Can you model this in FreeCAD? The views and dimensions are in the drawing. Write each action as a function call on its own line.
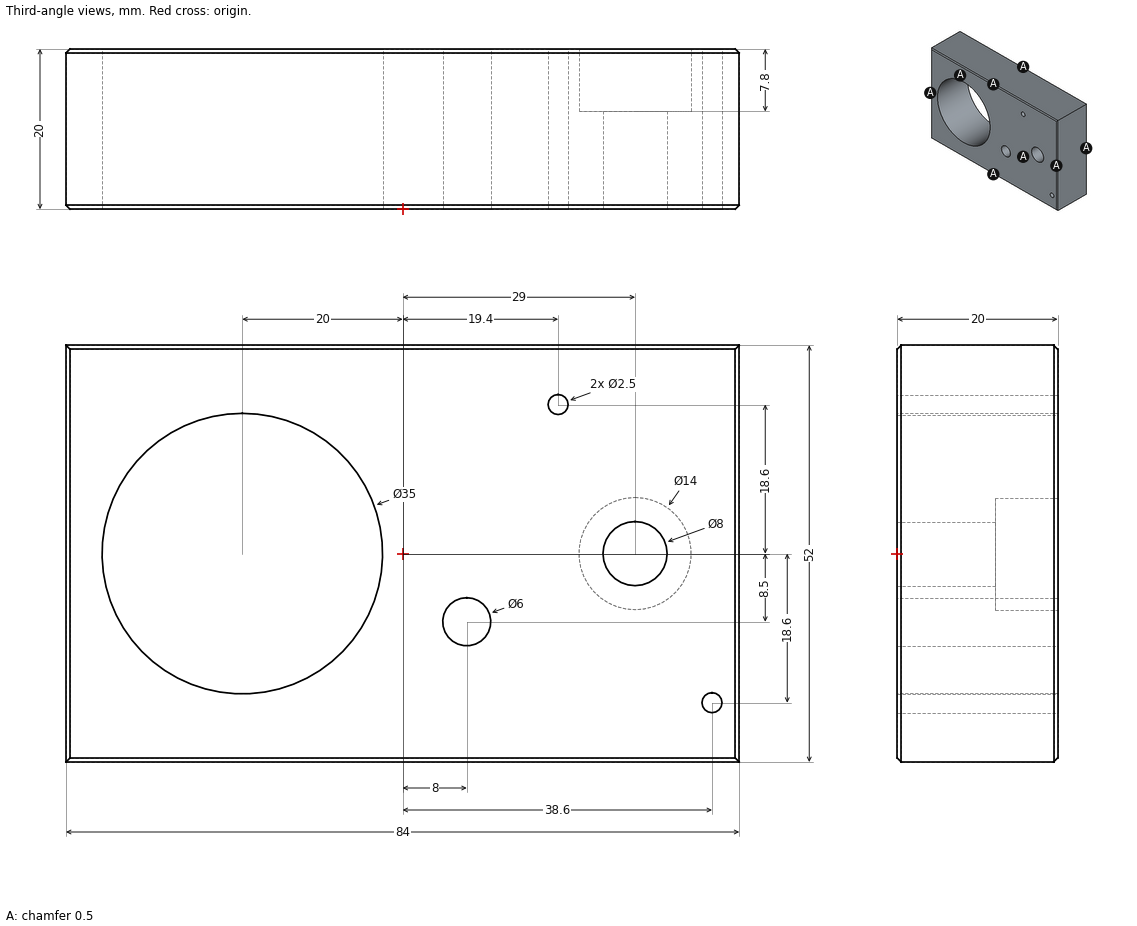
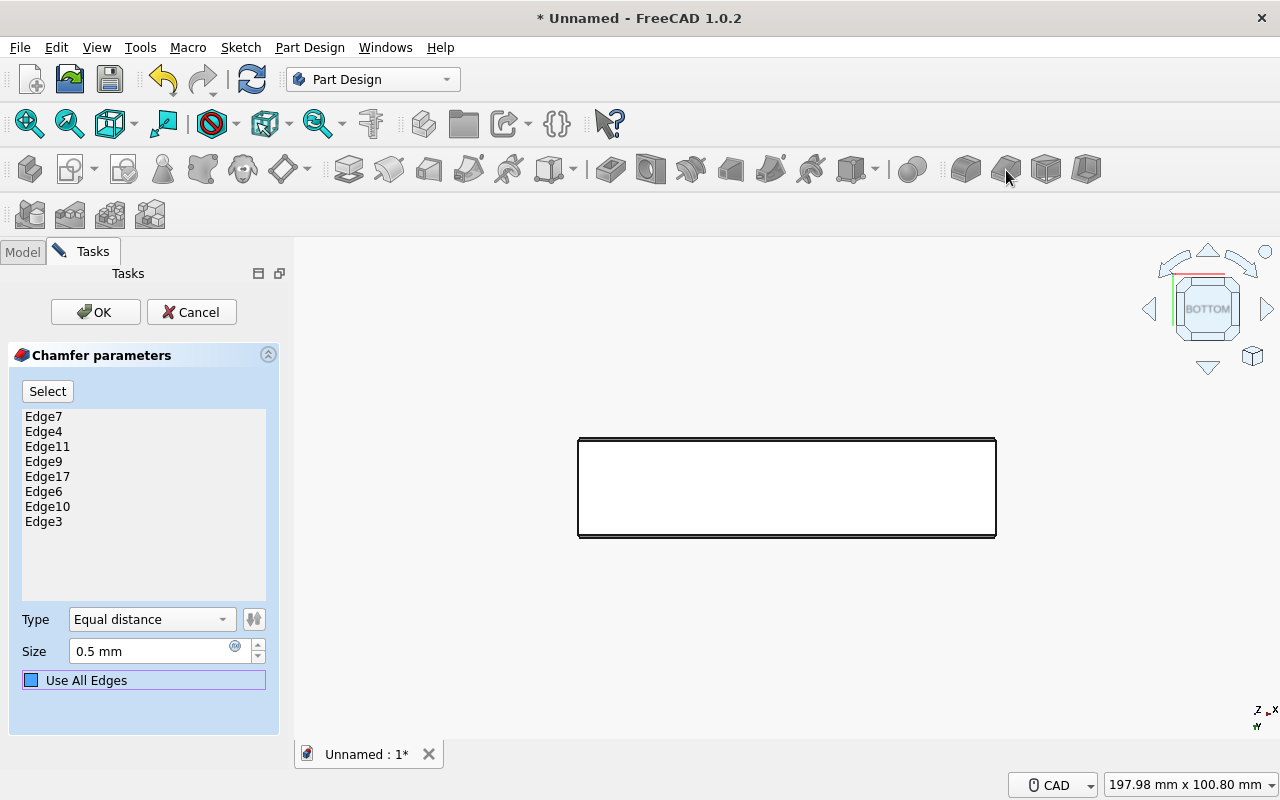
click(96, 312)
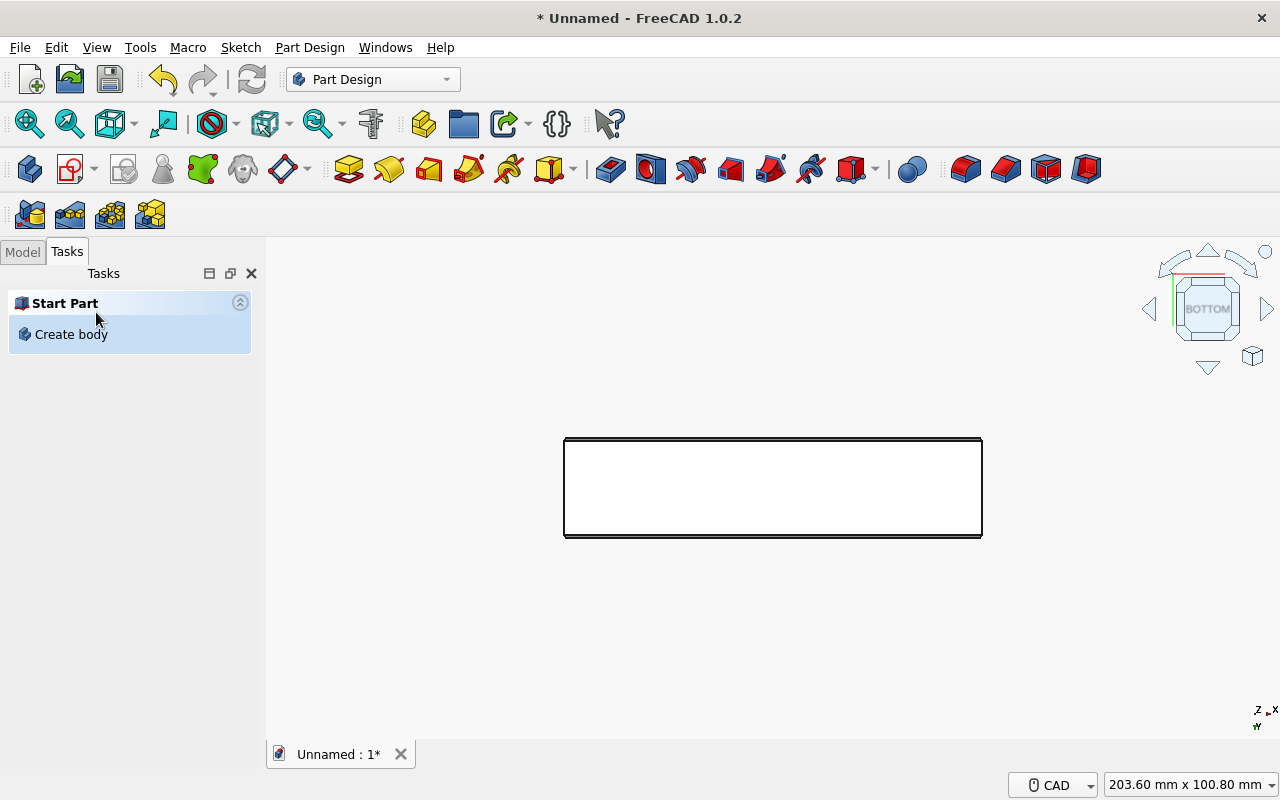
key(0)